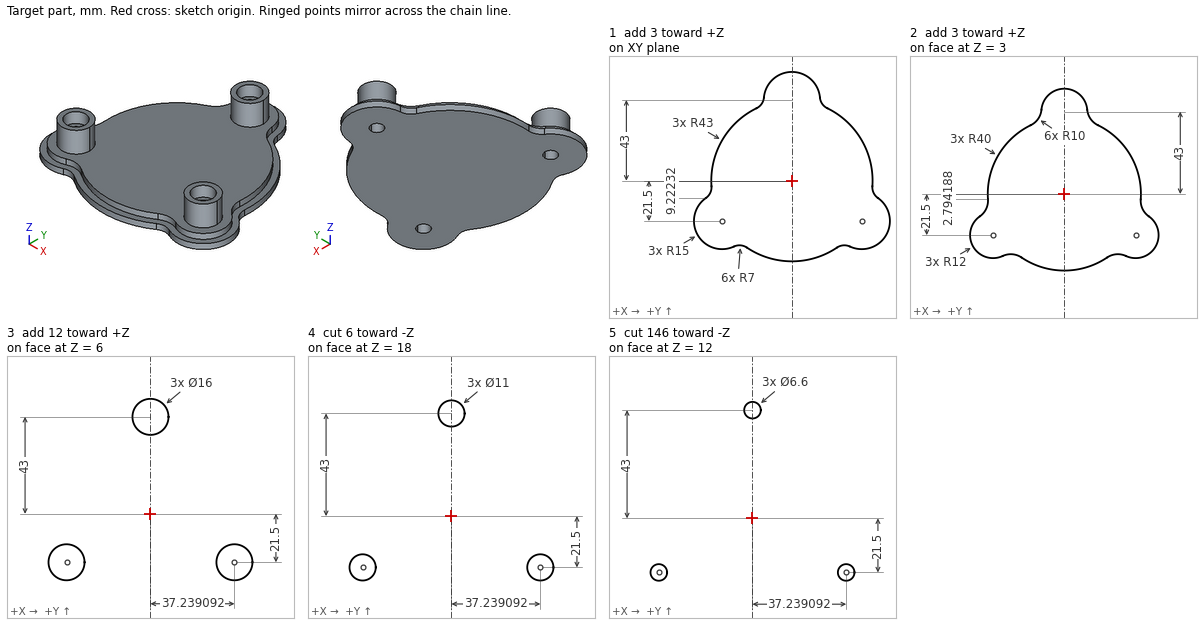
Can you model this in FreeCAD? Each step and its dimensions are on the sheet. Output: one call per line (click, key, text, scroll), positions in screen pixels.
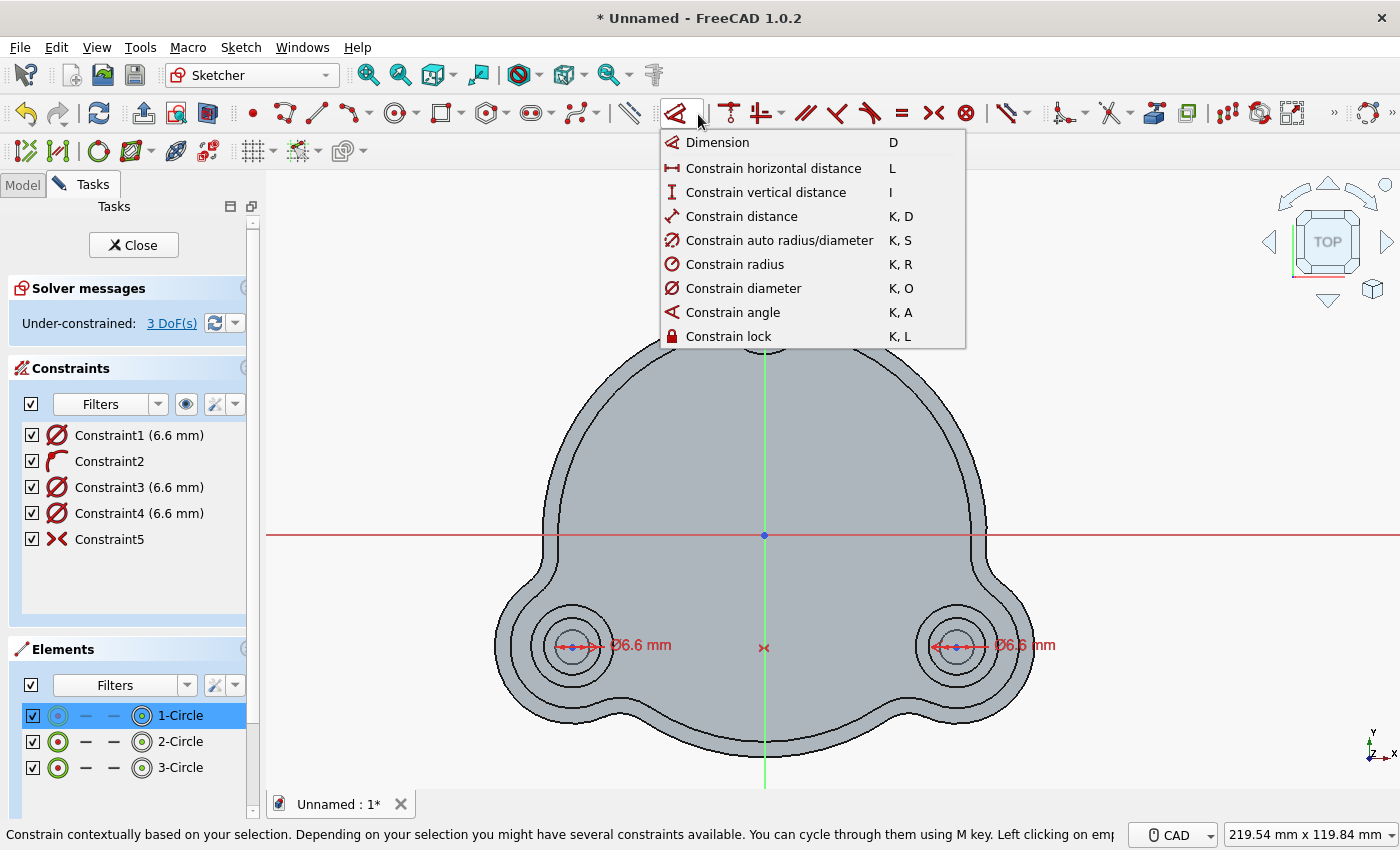
click(813, 192)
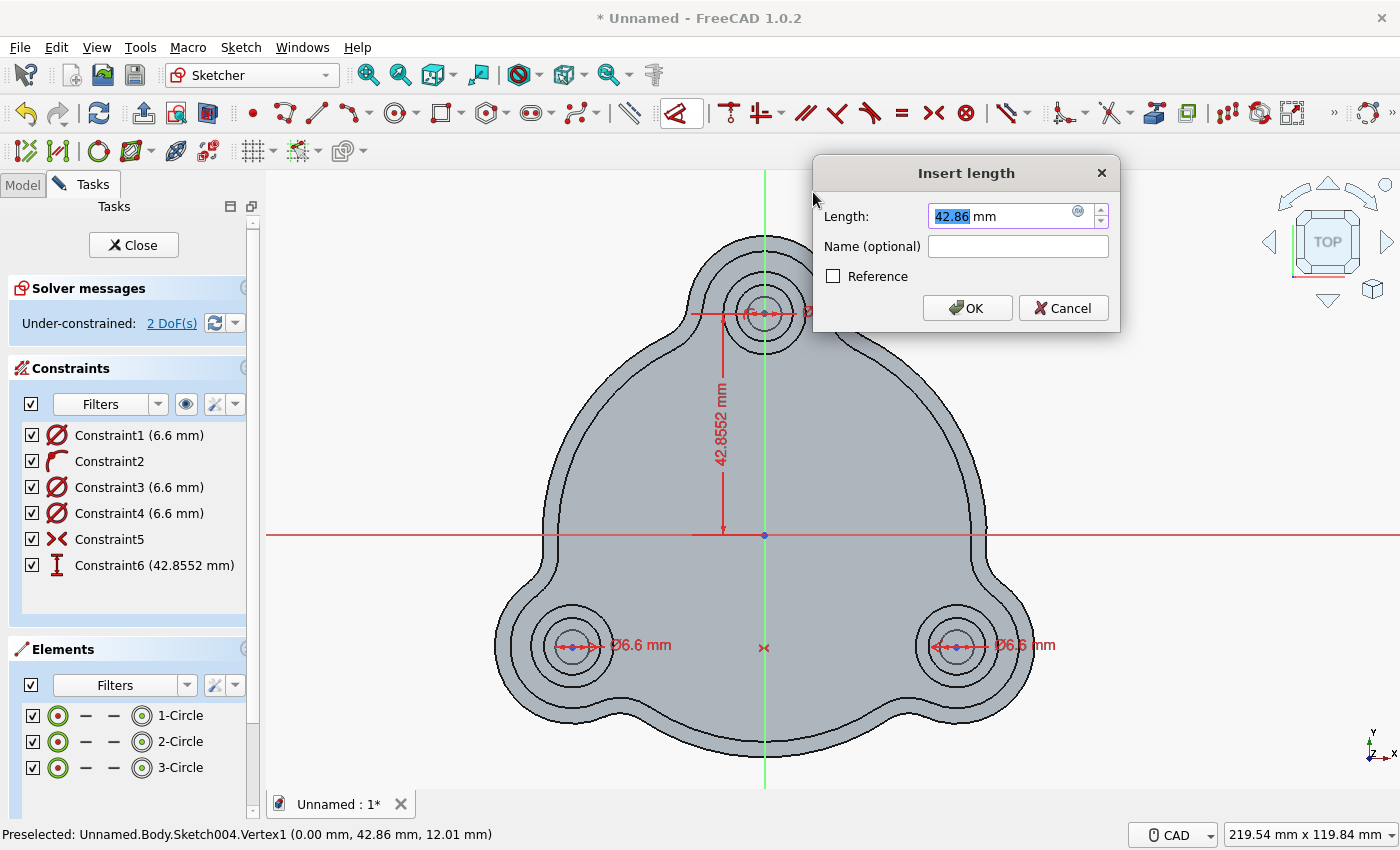
text(43)
key(Return)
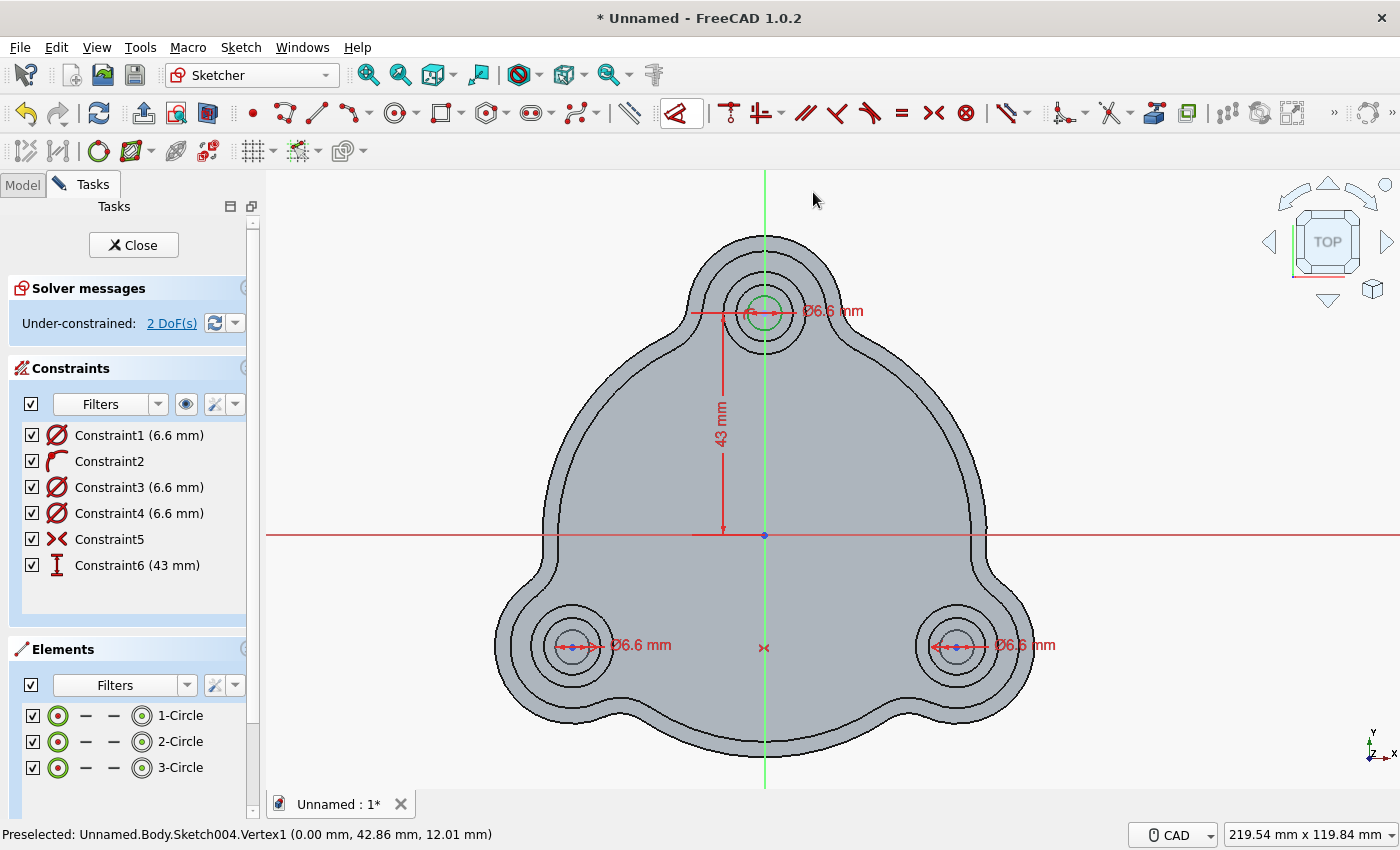
click(957, 647)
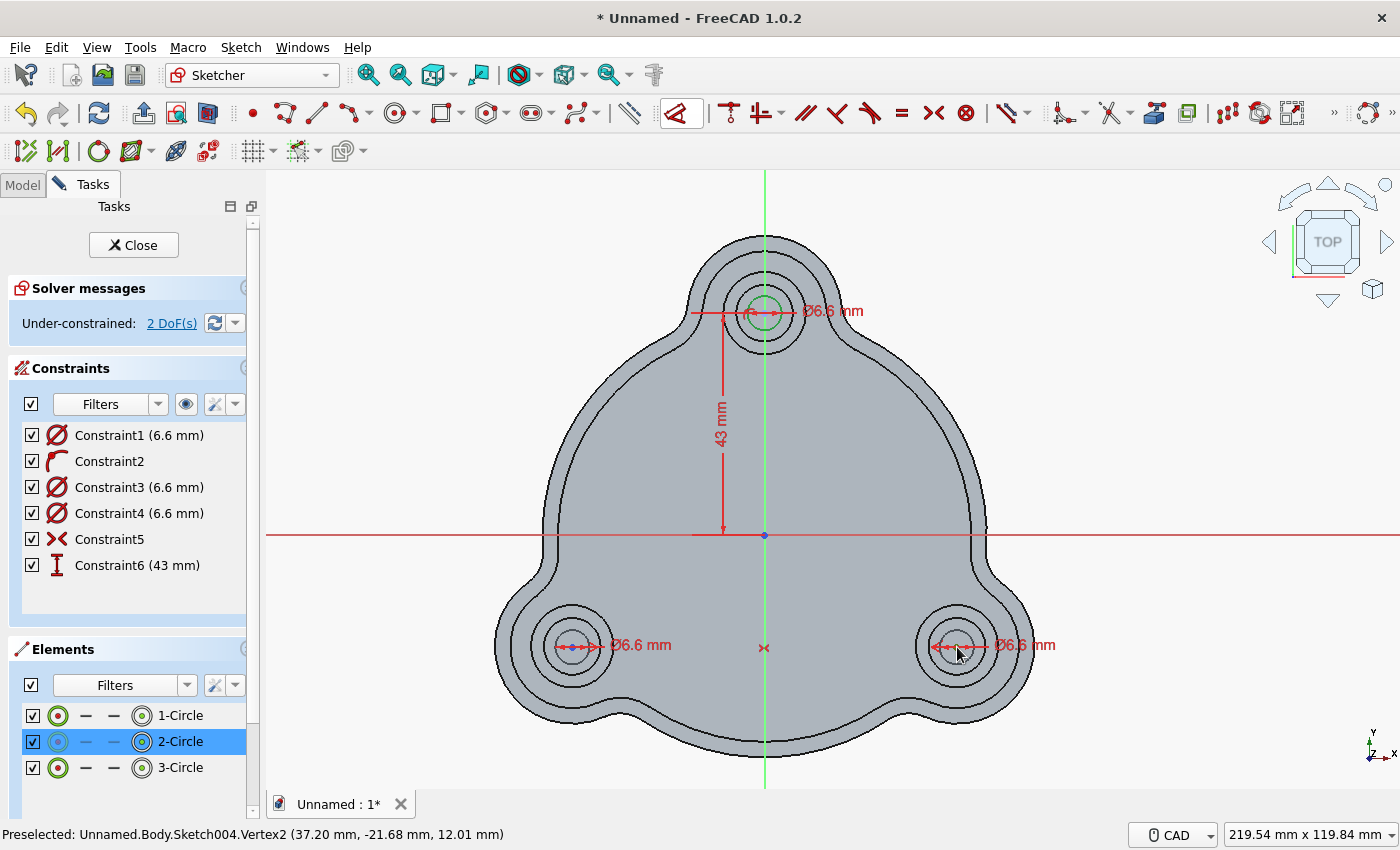
click(698, 114)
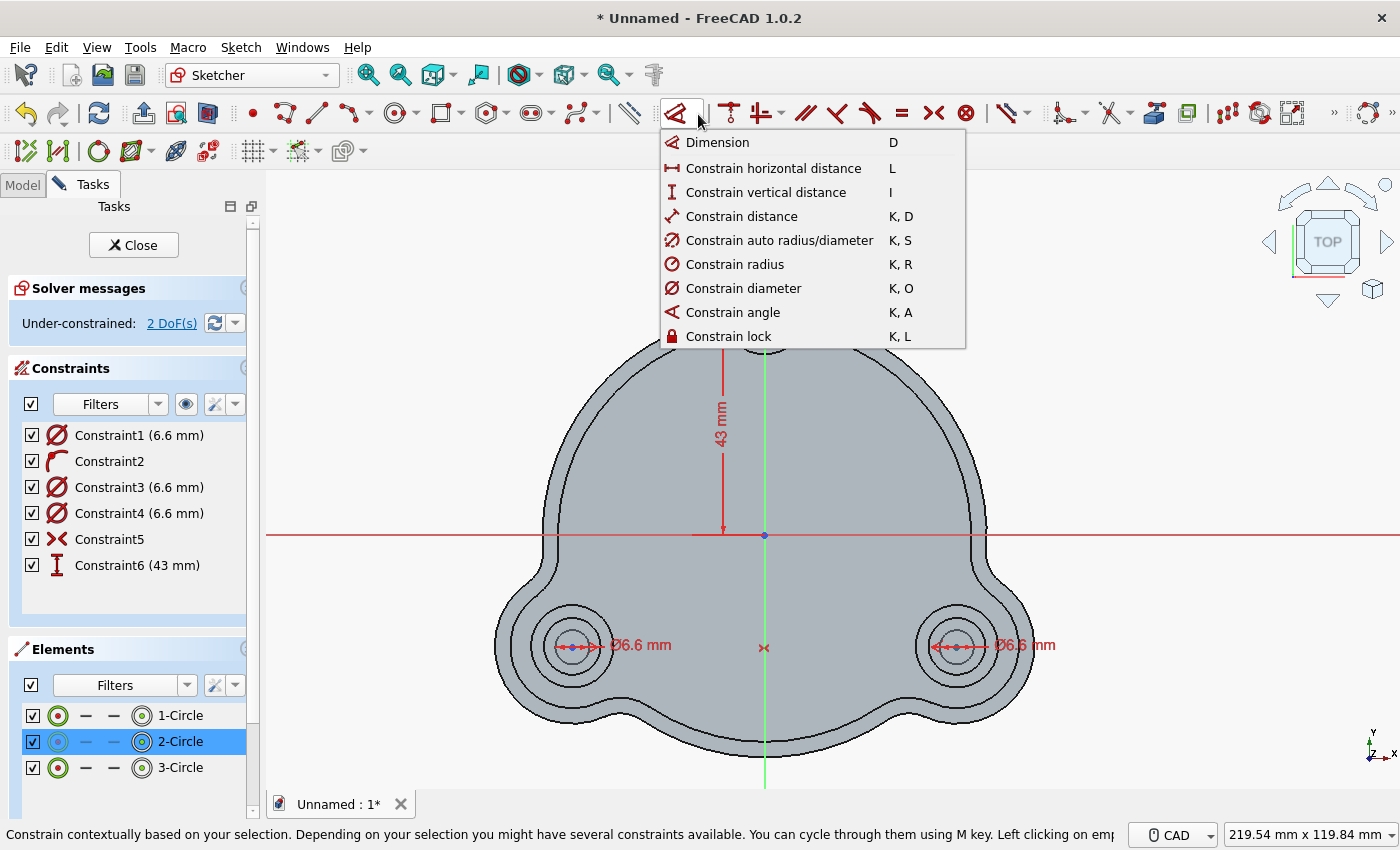
click(813, 192)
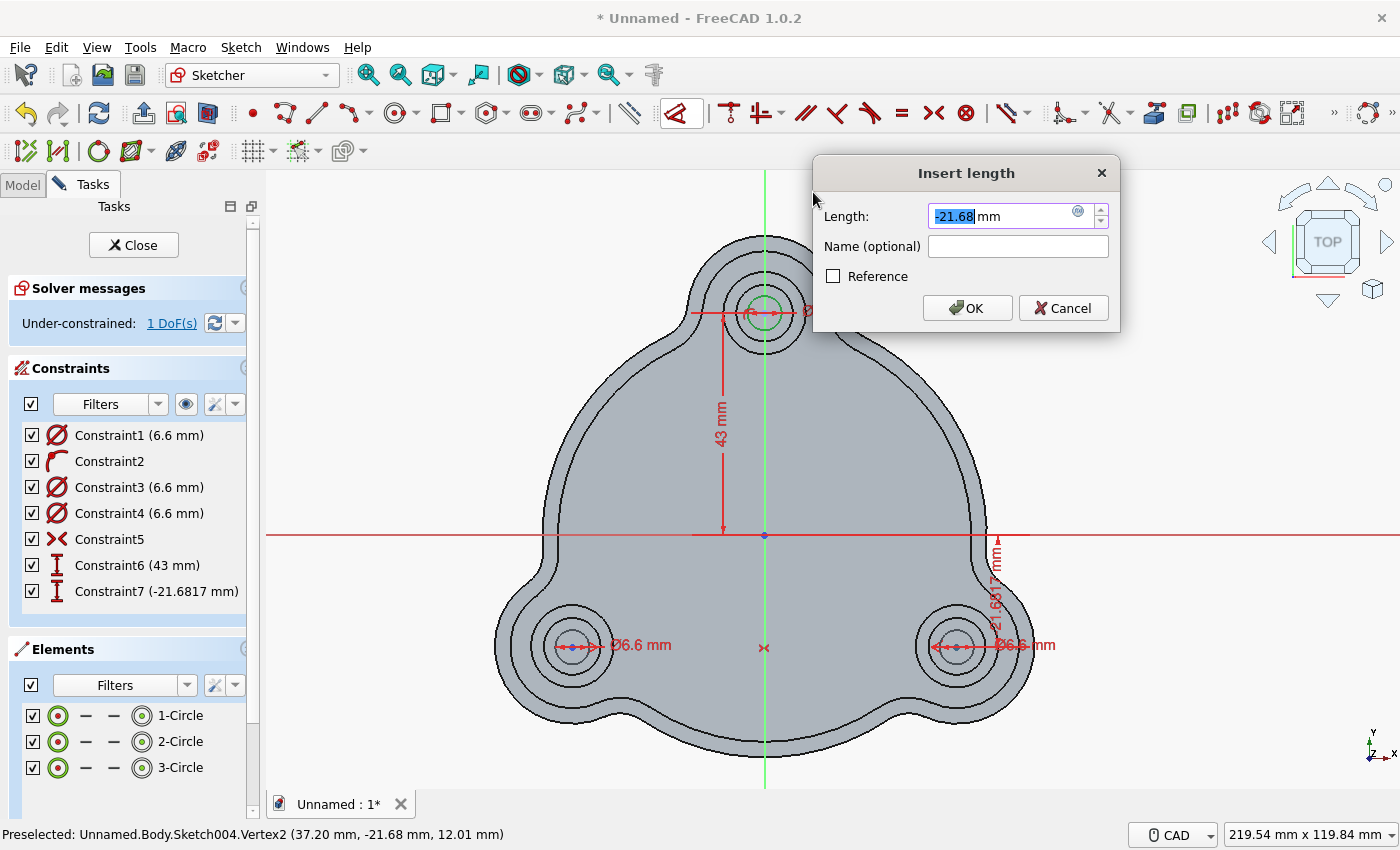
text(-21.5)
key(Return)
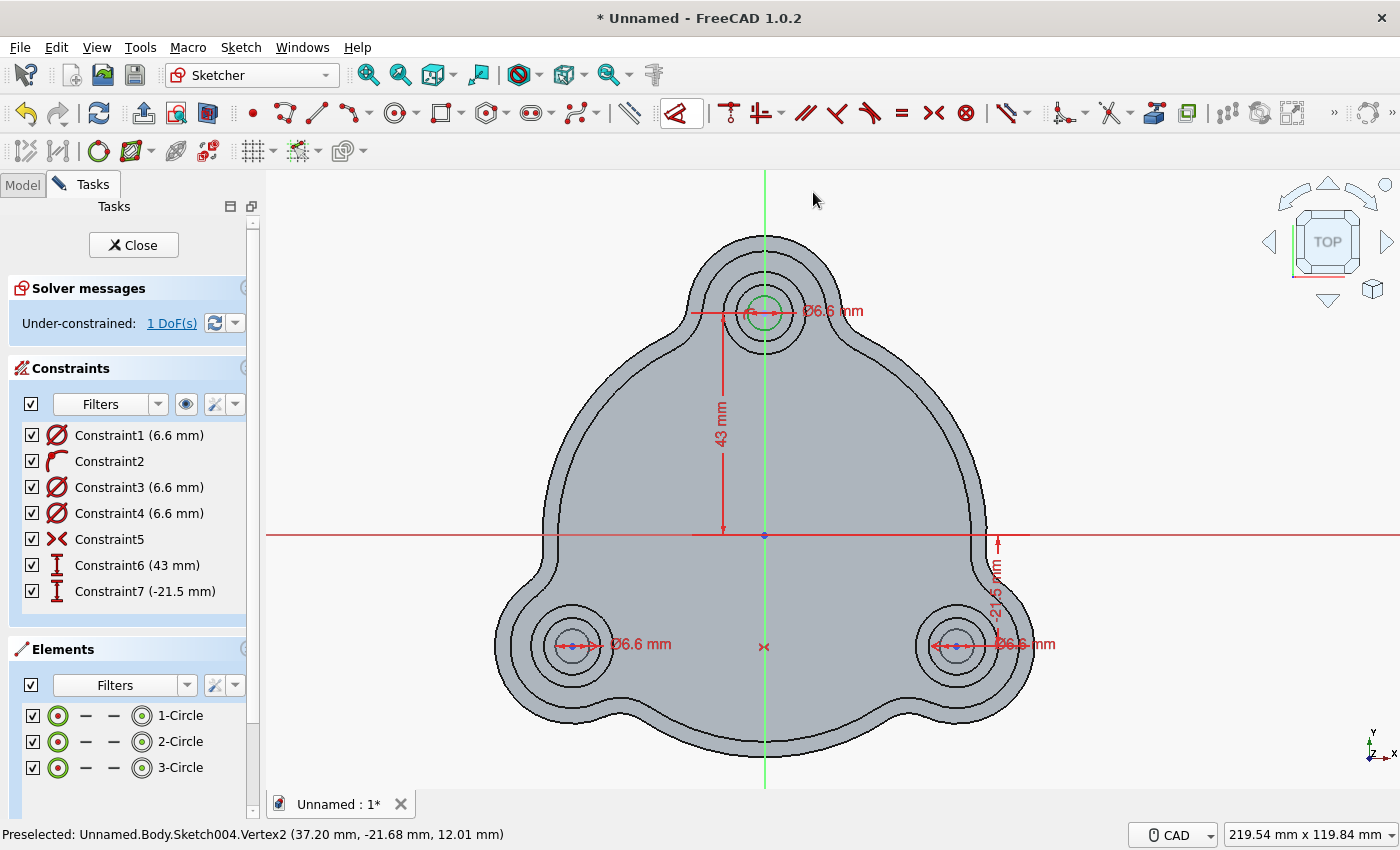
click(957, 646)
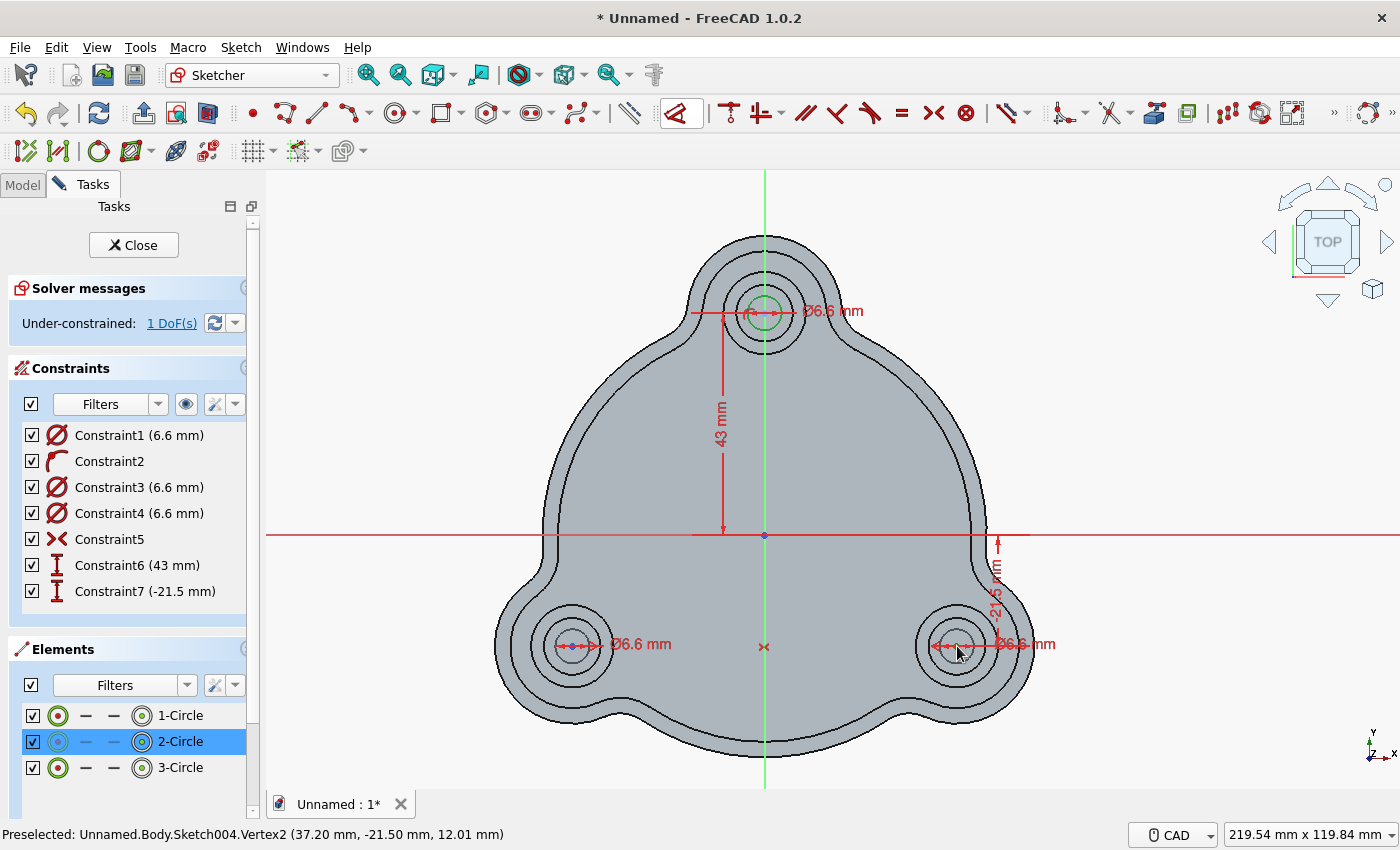
key(l)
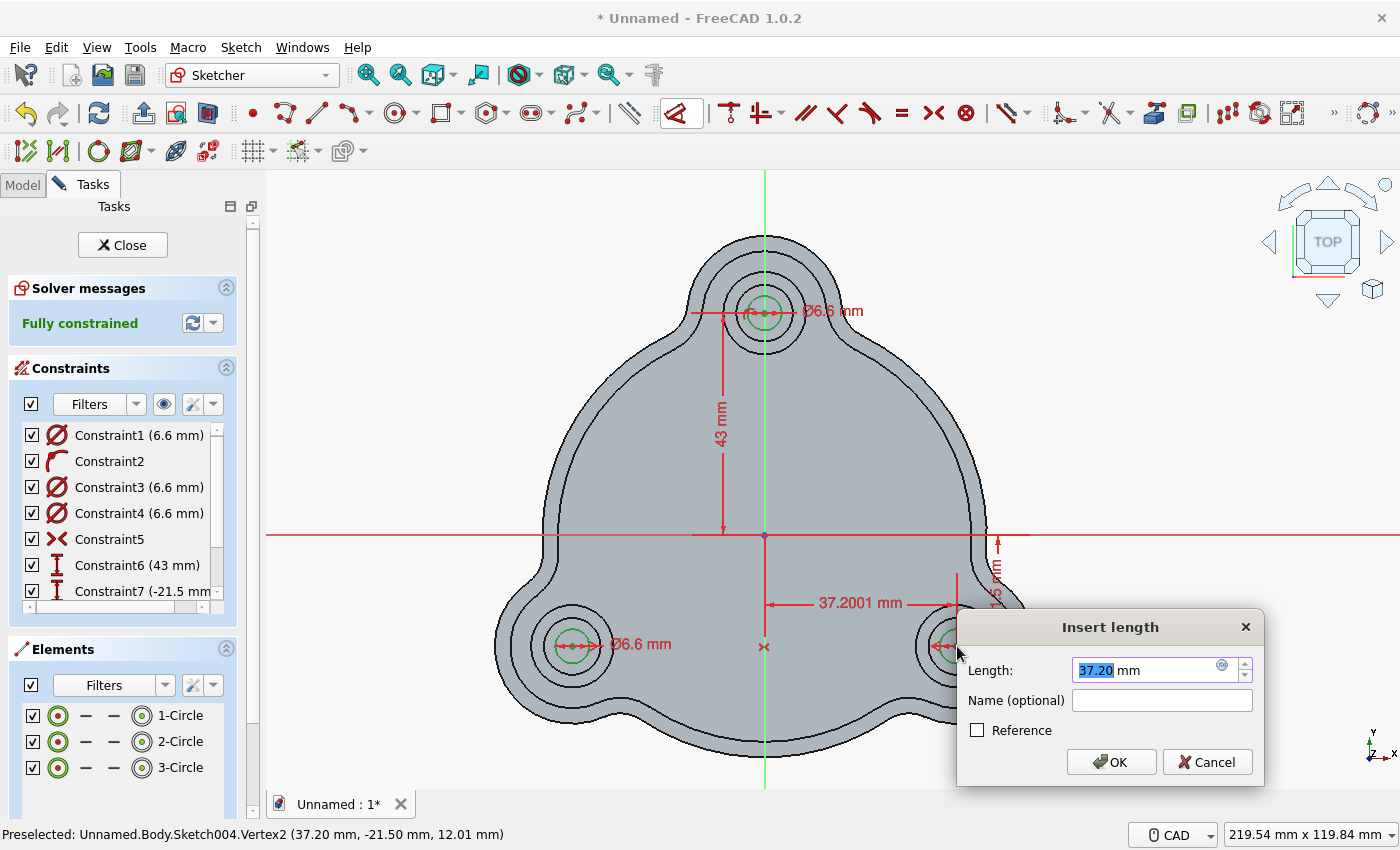
text(37.239092)
key(Return)